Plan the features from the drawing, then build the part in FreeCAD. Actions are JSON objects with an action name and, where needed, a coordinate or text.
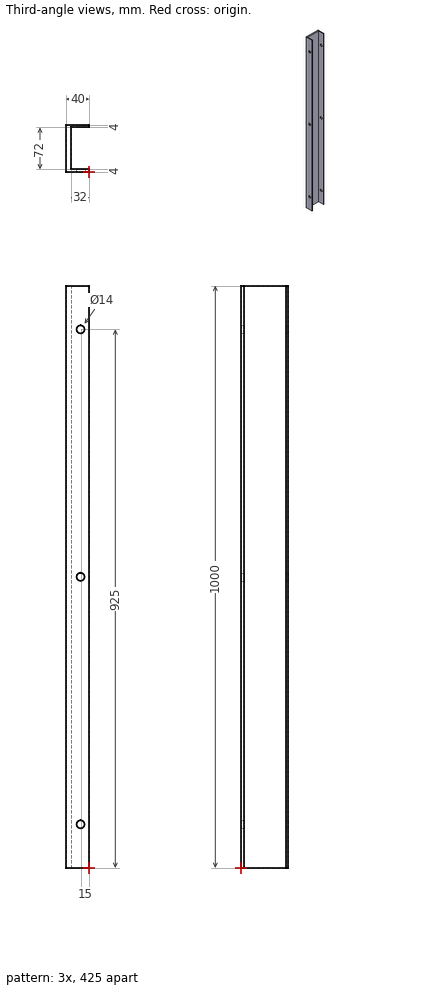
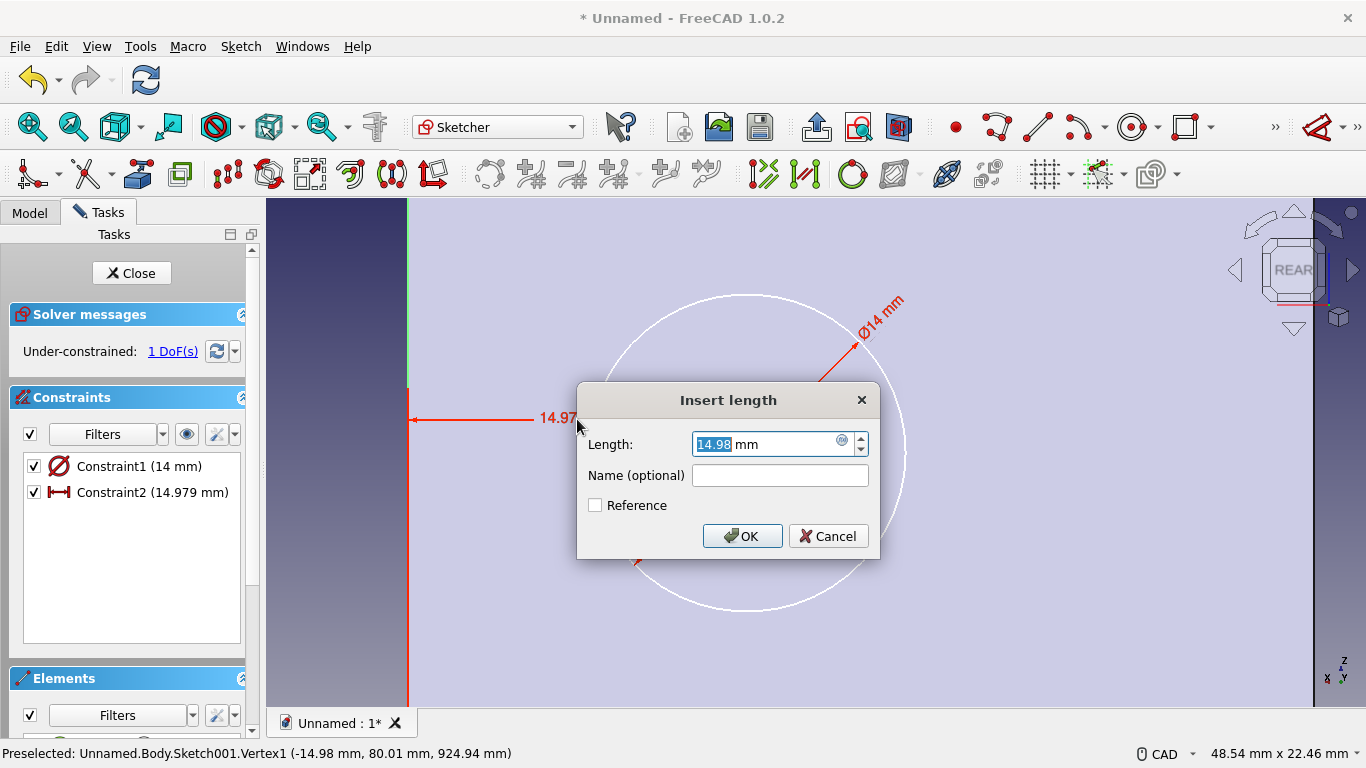
{"action": "type", "text": "15"}
{"action": "key", "text": "Return"}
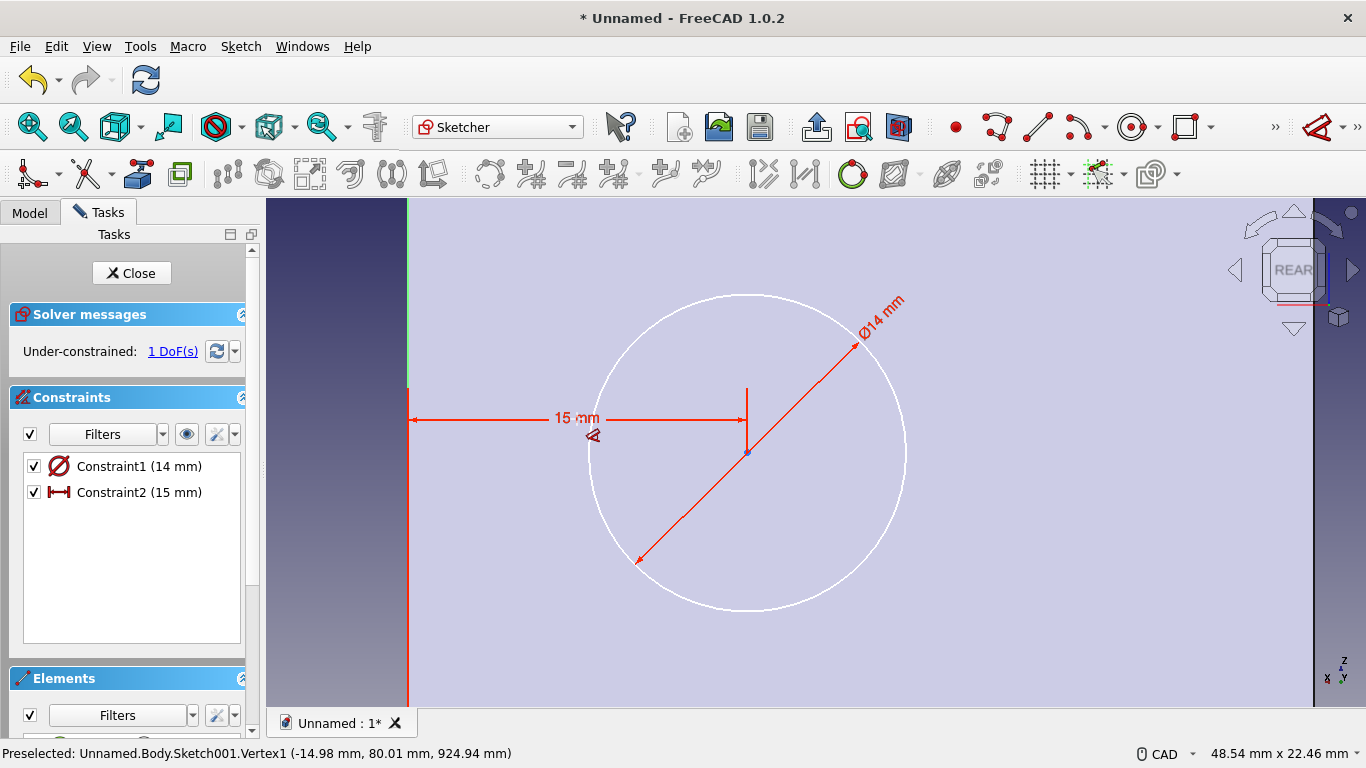
{"action": "left_click", "coordinate": [747, 453]}
{"action": "left_click", "coordinate": [374, 566]}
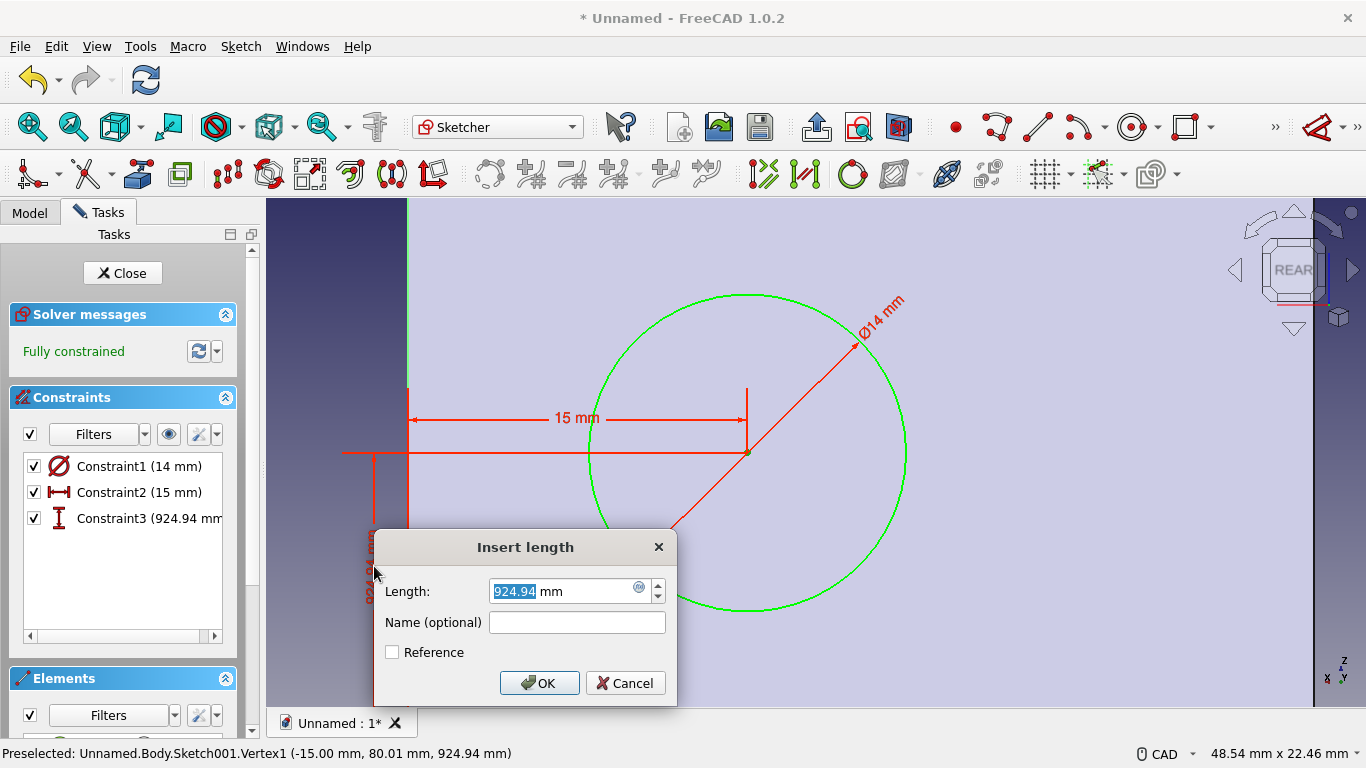
{"action": "type", "text": "925"}
{"action": "key", "text": "Return"}
{"action": "key", "text": "Escape"}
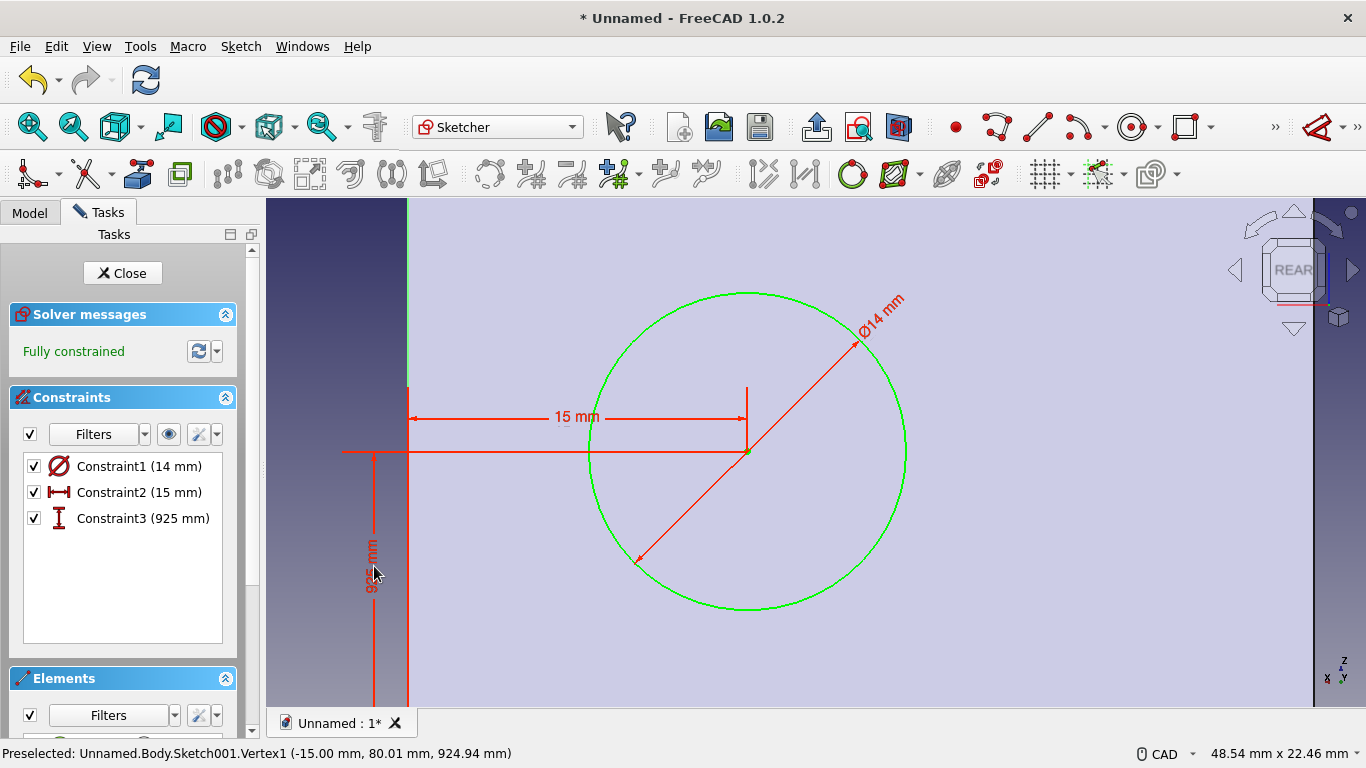
{"action": "left_click", "coordinate": [123, 273]}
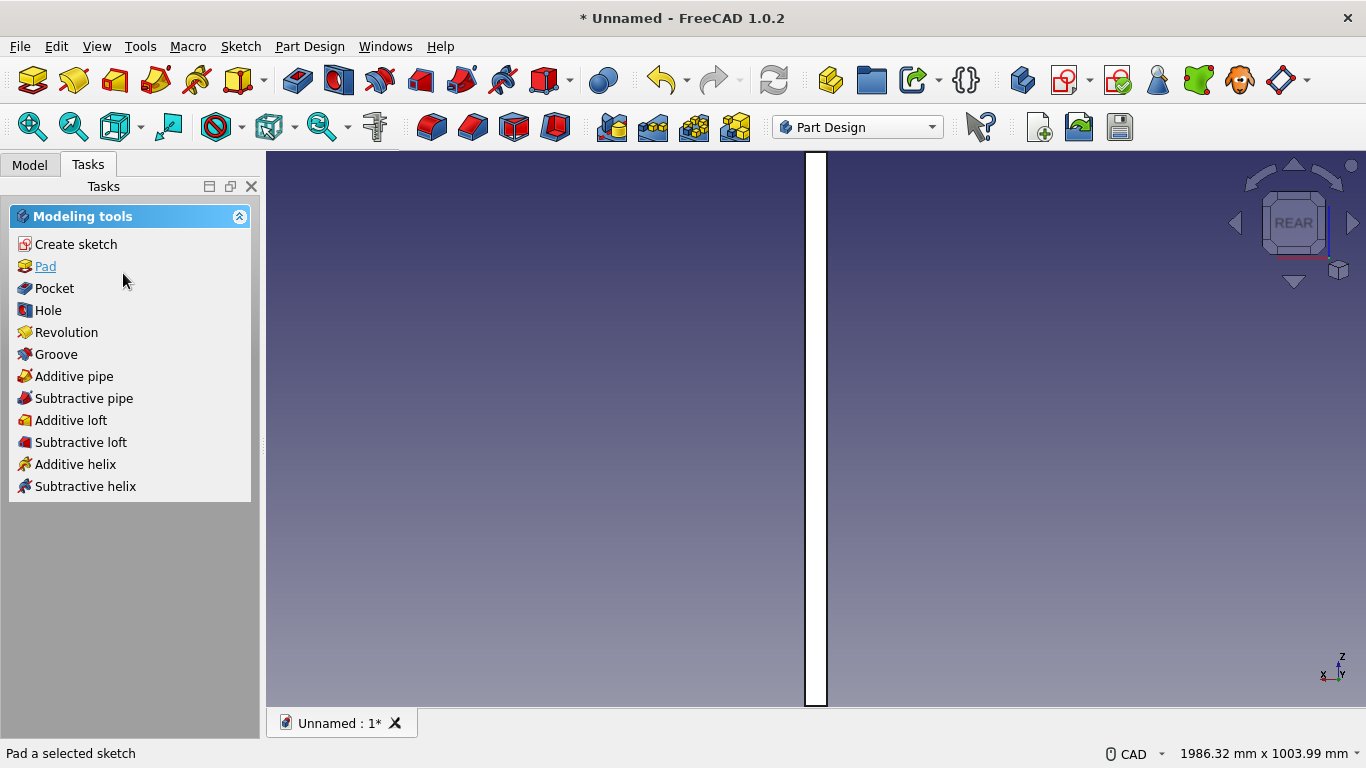
{"action": "left_click", "coordinate": [298, 80]}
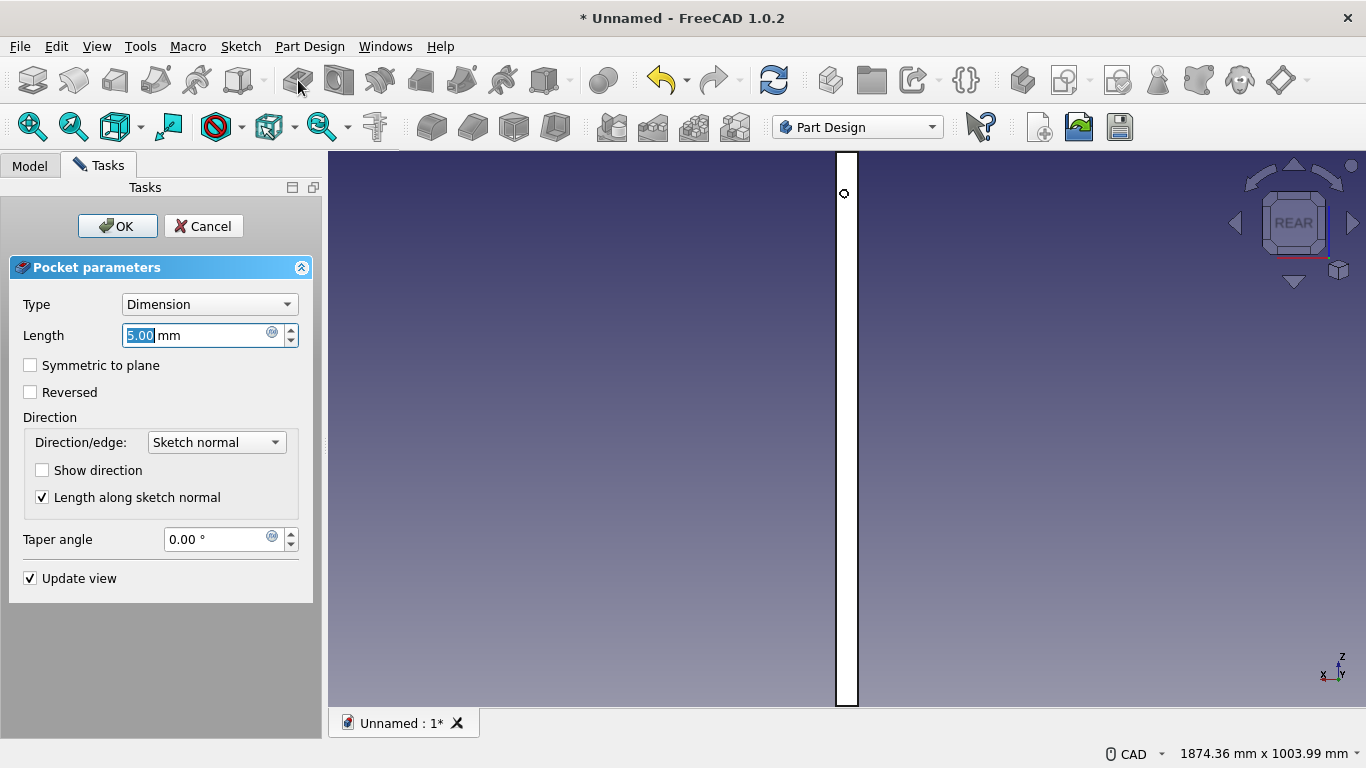
{"action": "left_click", "coordinate": [210, 304]}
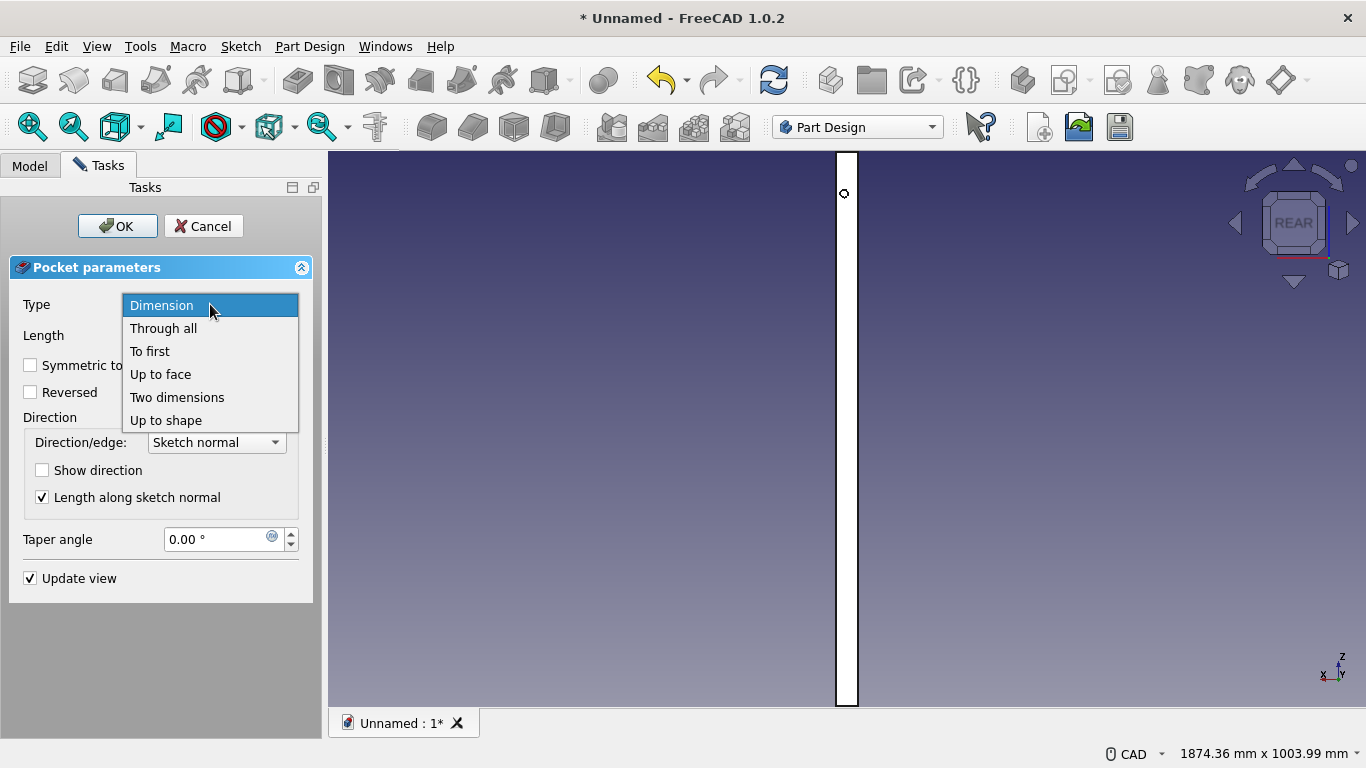
{"action": "left_click", "coordinate": [208, 328]}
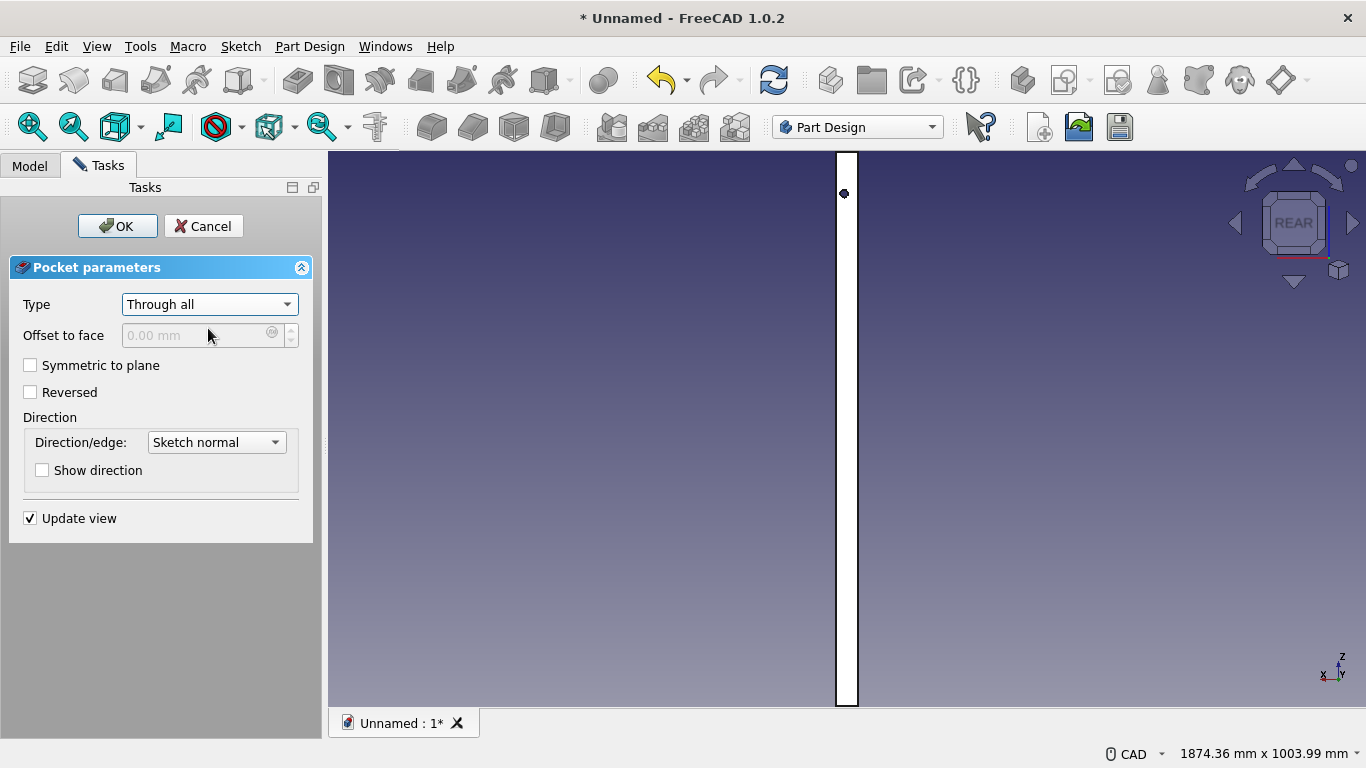
{"action": "left_click", "coordinate": [118, 226]}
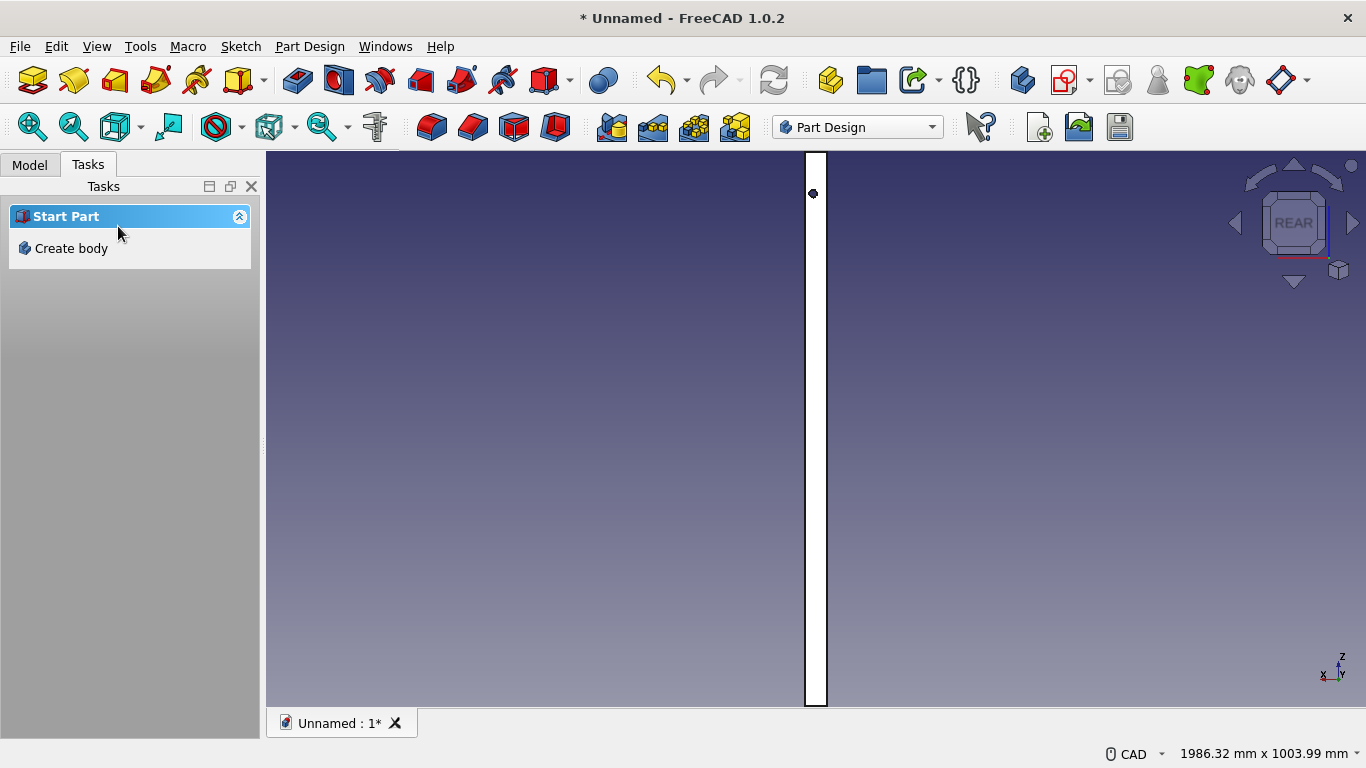
{"action": "left_click", "coordinate": [30, 164]}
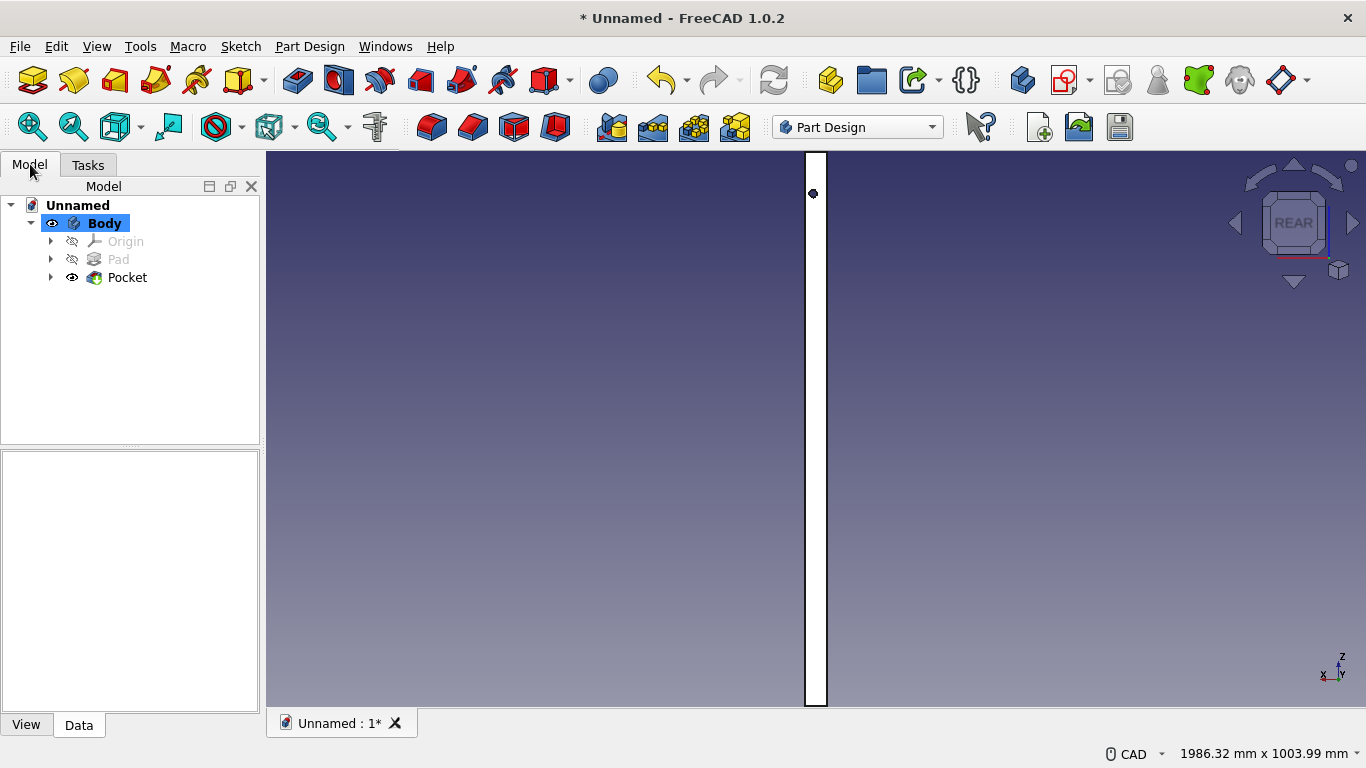
{"action": "left_click", "coordinate": [117, 277]}